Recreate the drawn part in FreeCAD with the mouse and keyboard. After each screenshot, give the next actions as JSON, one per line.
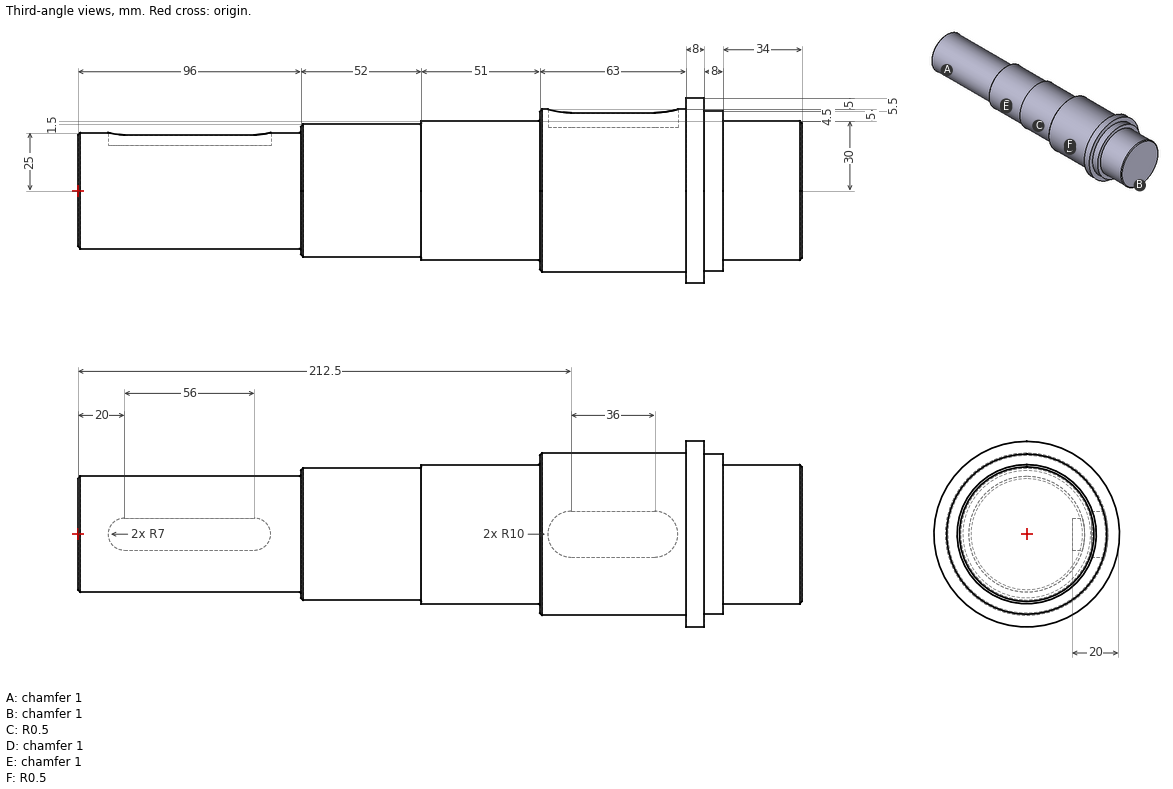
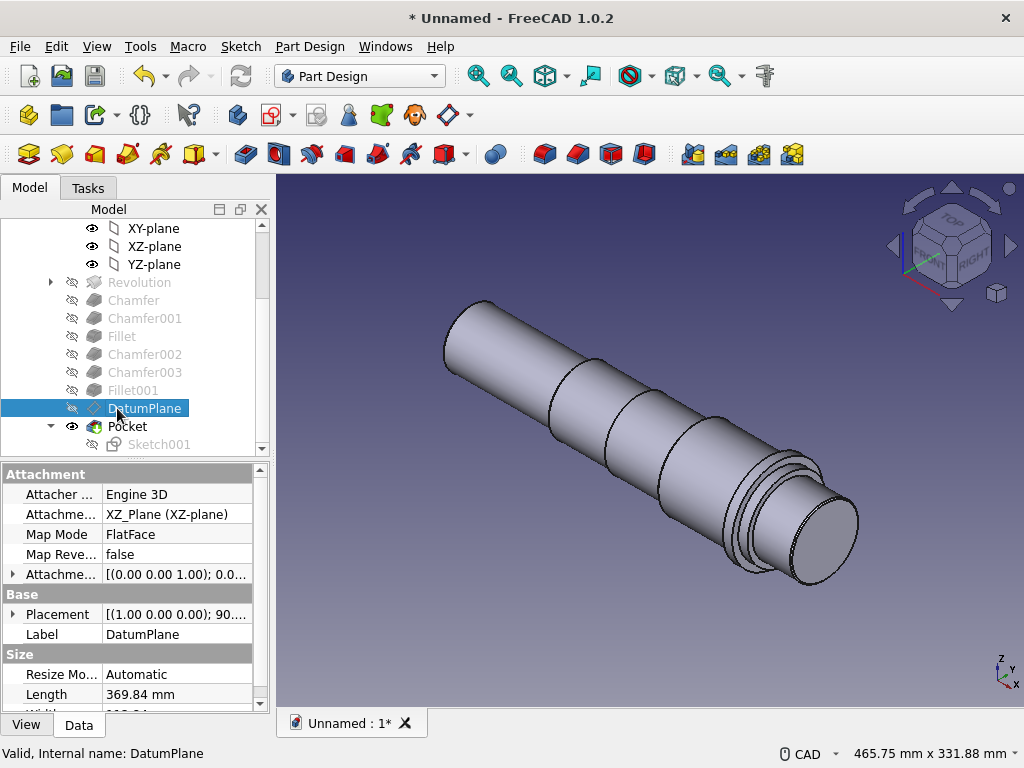
{"action": "scroll", "coordinate": [161, 332], "scroll_direction": "down", "scroll_amount": 3}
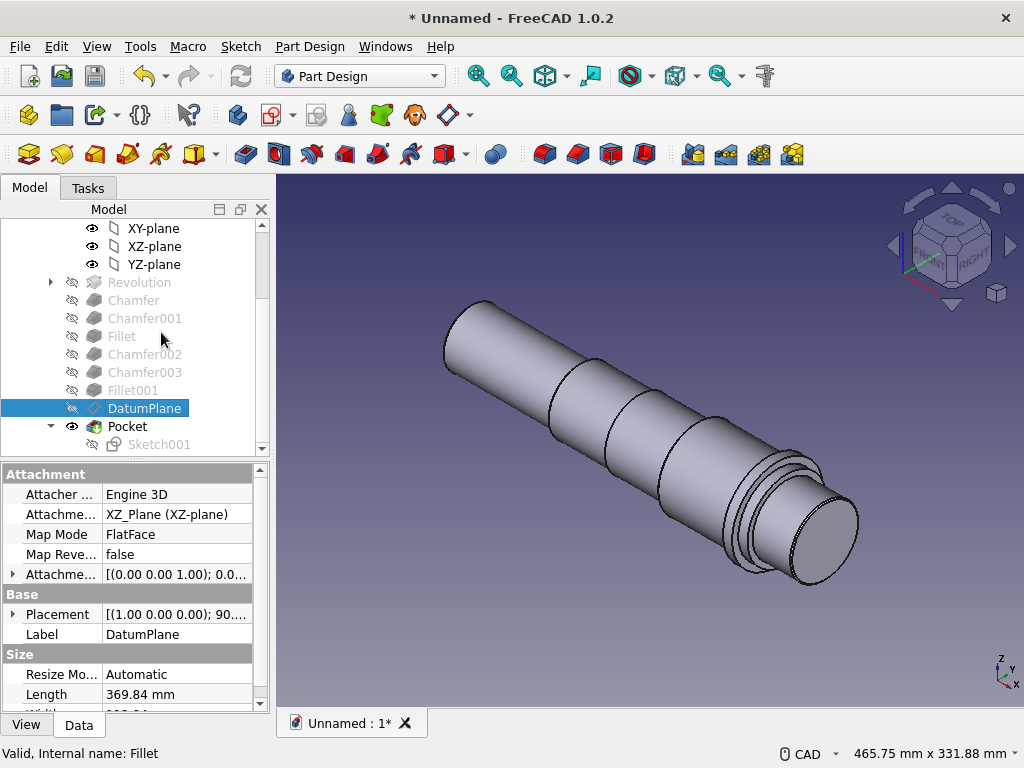
{"action": "scroll", "coordinate": [161, 332], "scroll_direction": "up", "scroll_amount": 15}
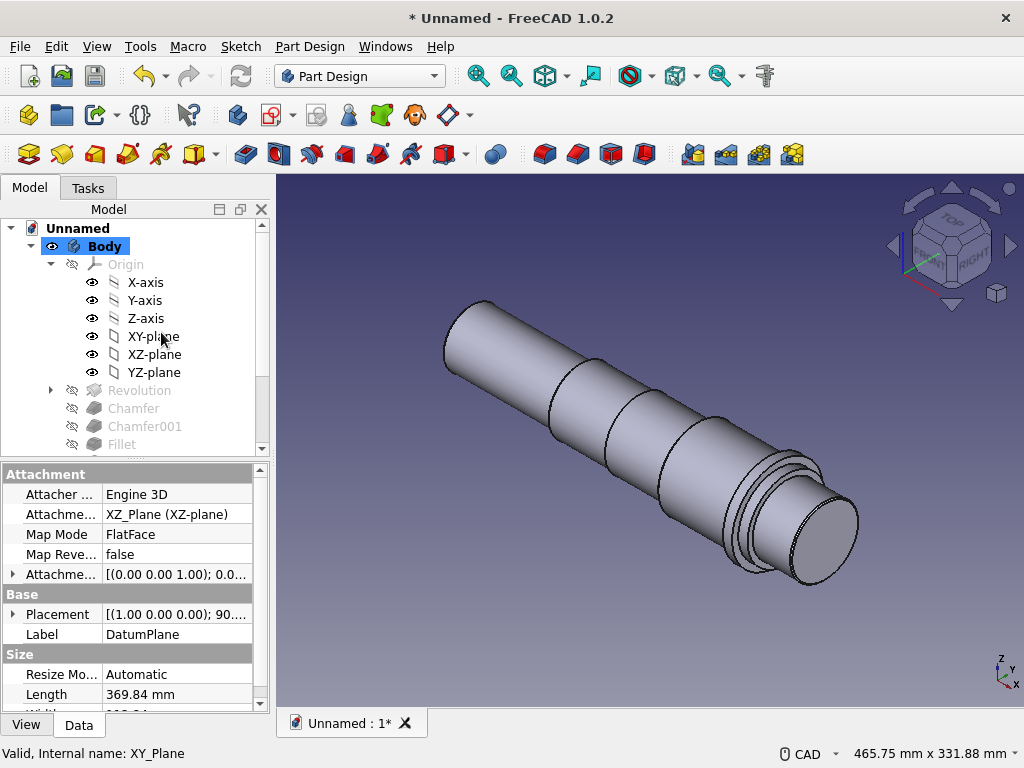
{"action": "left_click", "coordinate": [137, 354]}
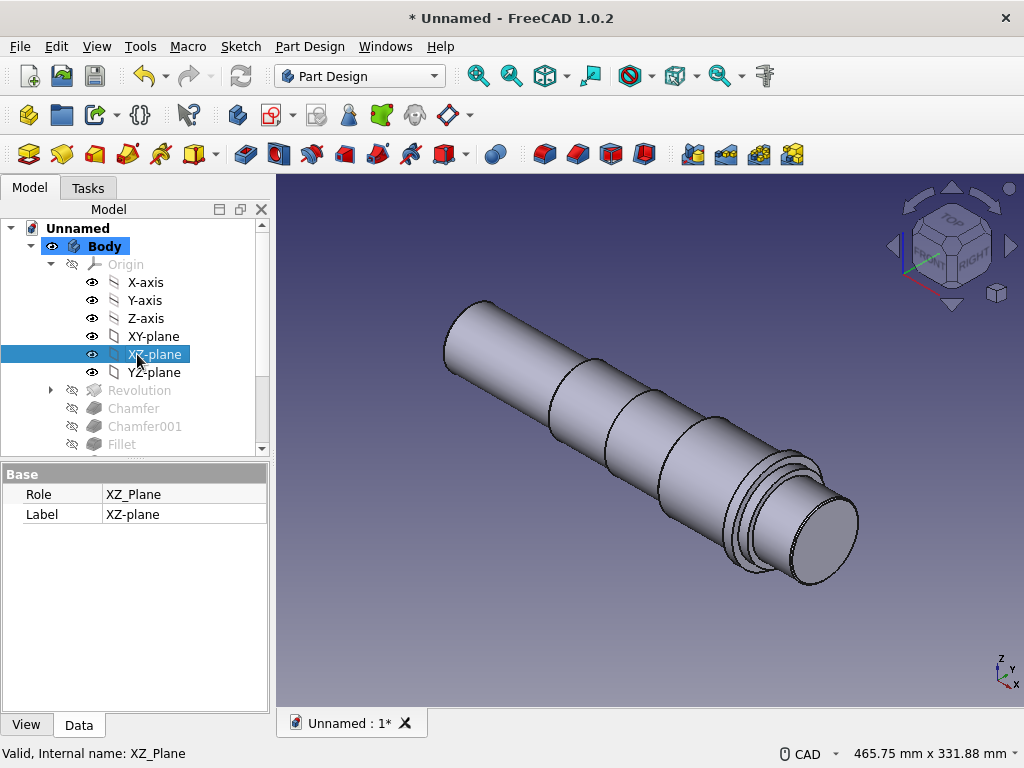
{"action": "left_click", "coordinate": [448, 116]}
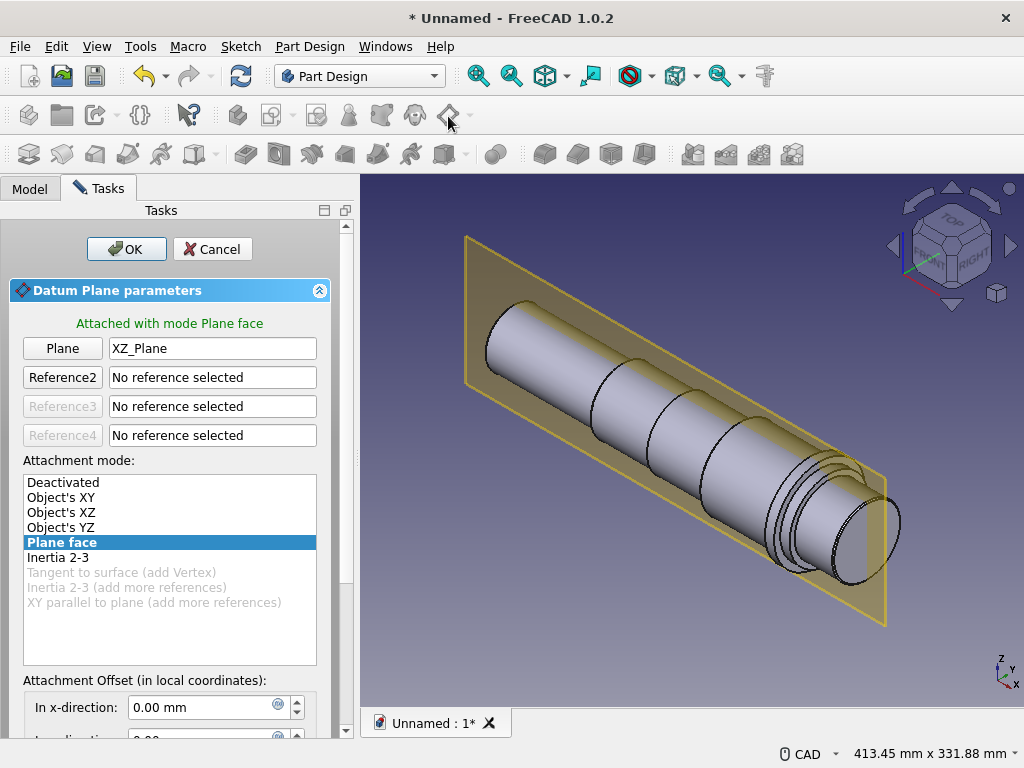
{"action": "scroll", "coordinate": [346, 479], "scroll_direction": "down", "scroll_amount": 2}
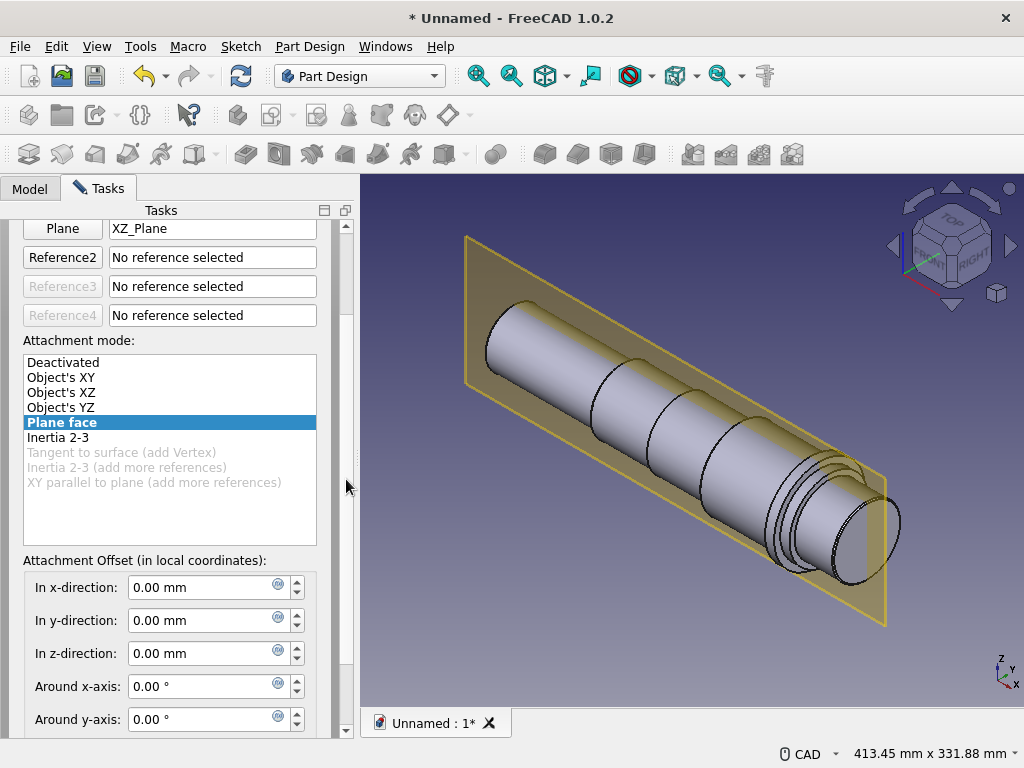
{"action": "triple_click", "coordinate": [210, 654]}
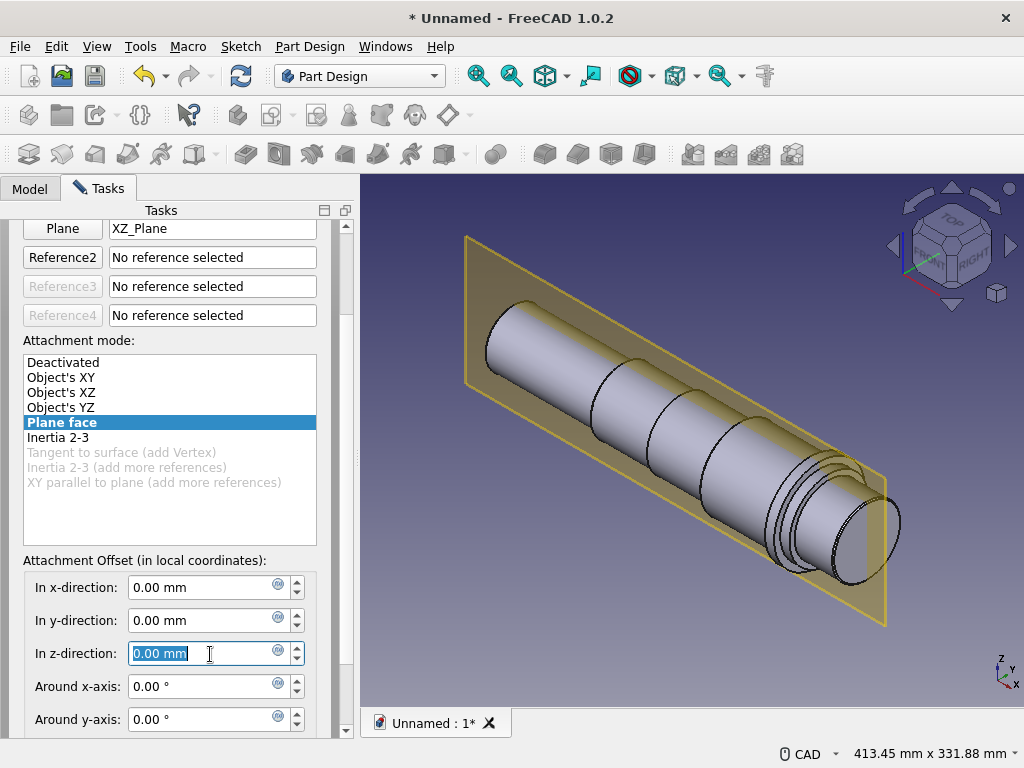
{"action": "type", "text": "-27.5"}
{"action": "key", "text": "Tab"}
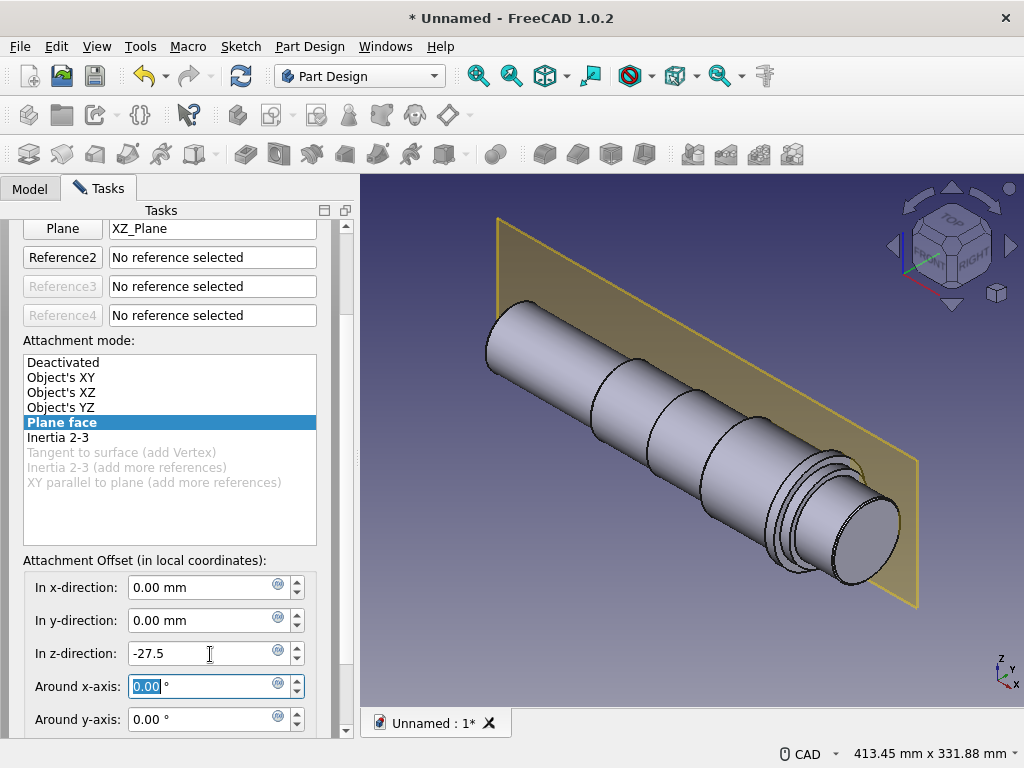
{"action": "scroll", "coordinate": [346, 479], "scroll_direction": "up", "scroll_amount": 3}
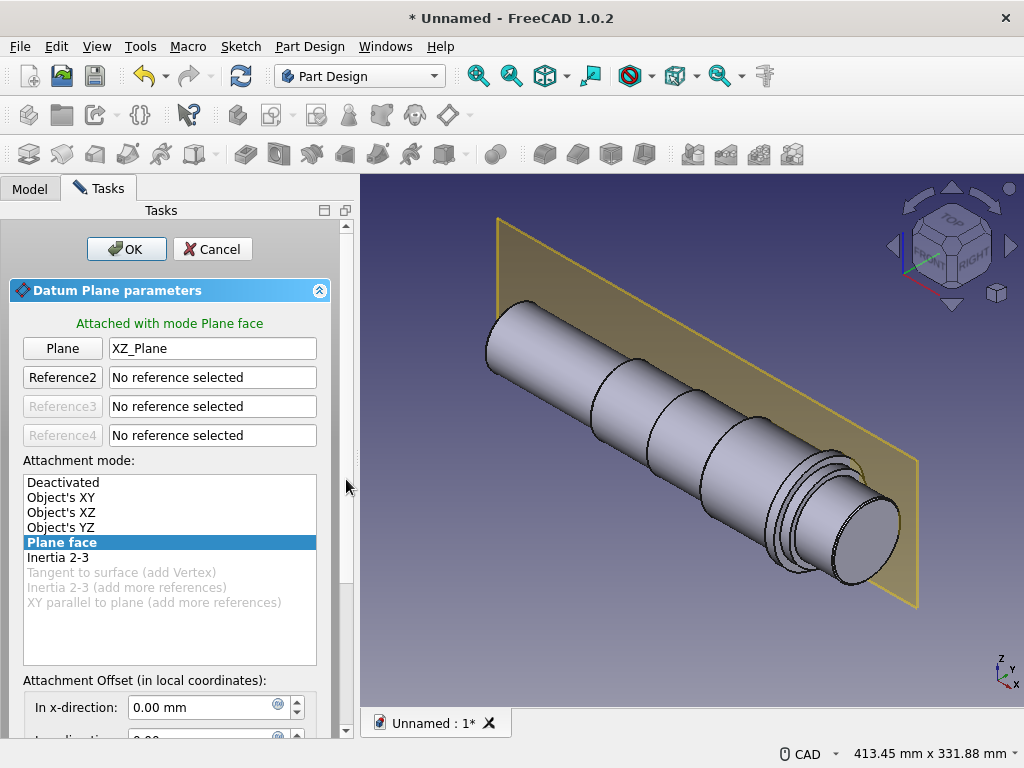
{"action": "left_click", "coordinate": [127, 249]}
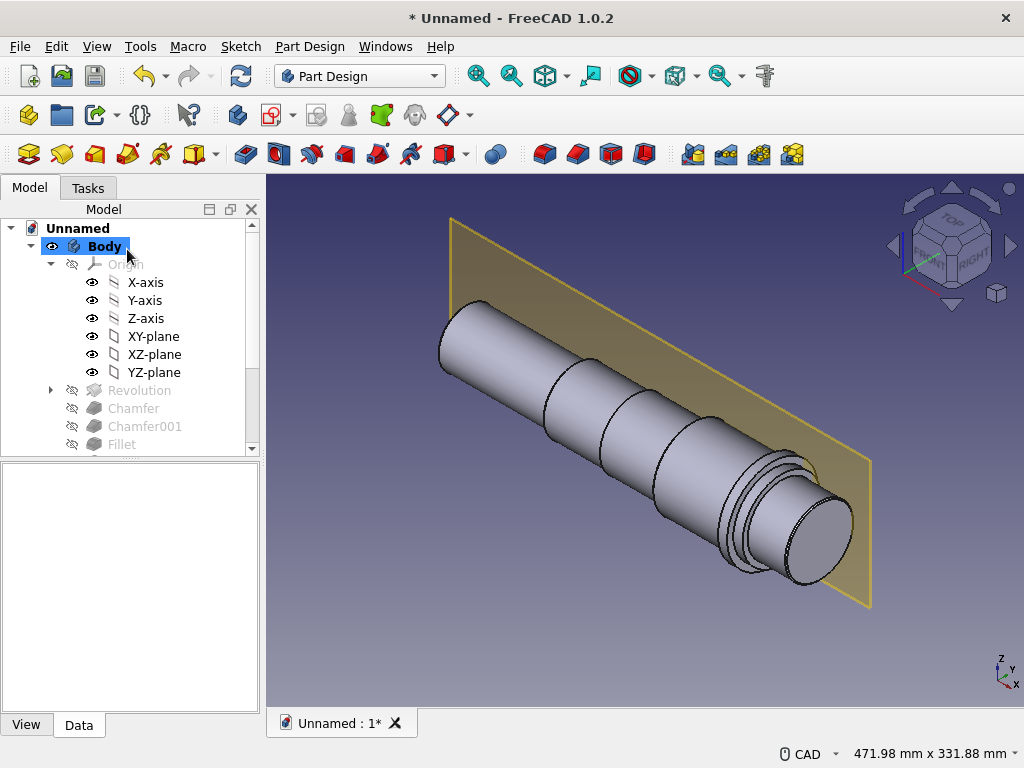
{"action": "scroll", "coordinate": [101, 332], "scroll_direction": "down", "scroll_amount": 3}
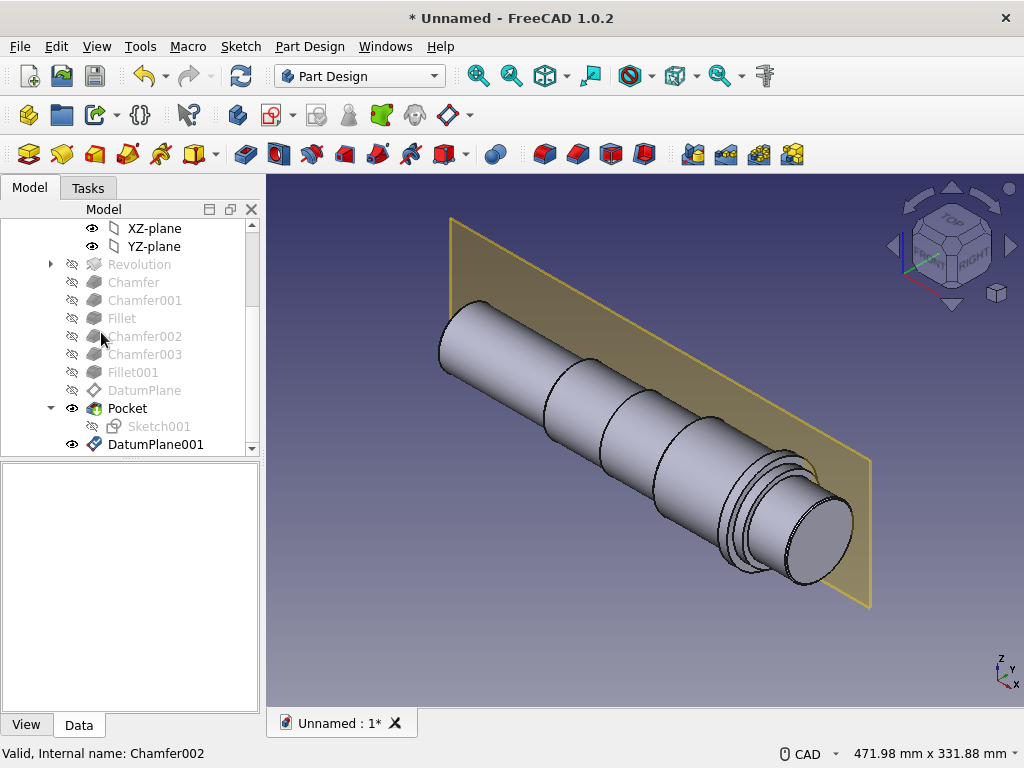
{"action": "left_click", "coordinate": [117, 444]}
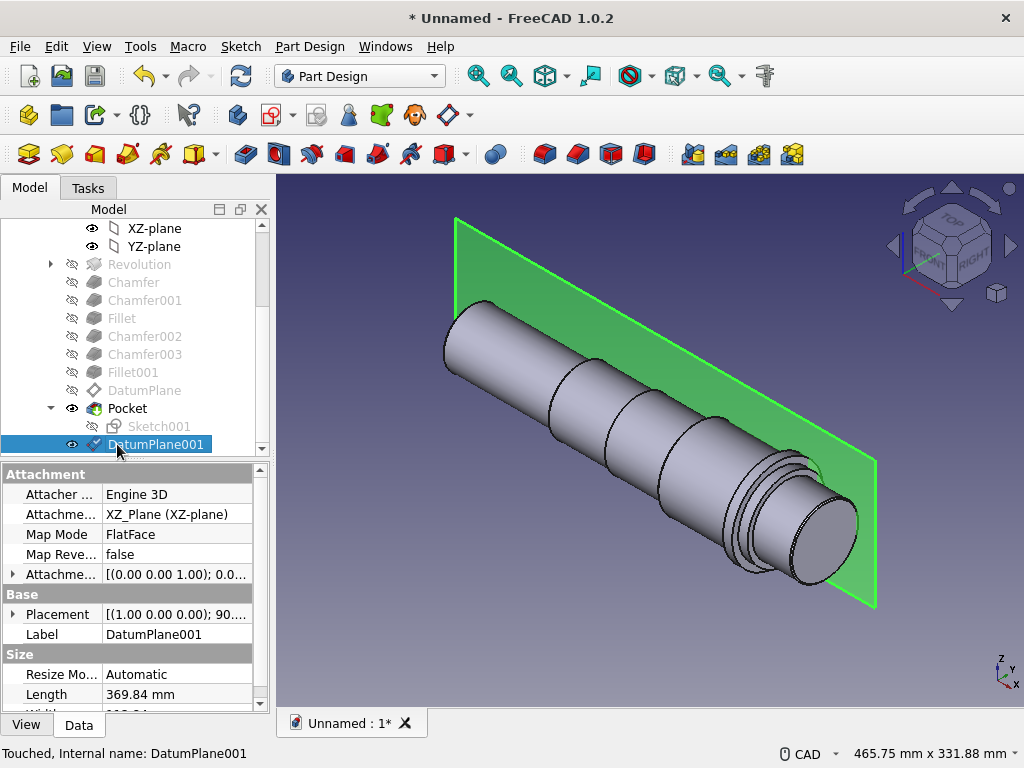
{"action": "left_click", "coordinate": [270, 116]}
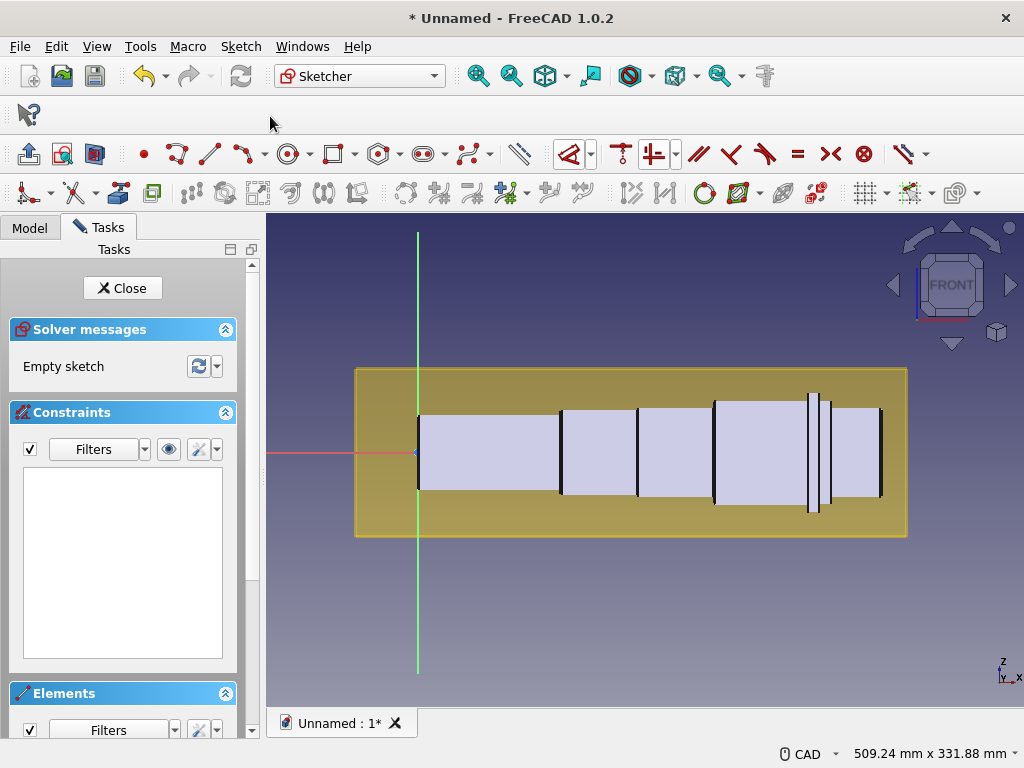
{"action": "left_click", "coordinate": [95, 154]}